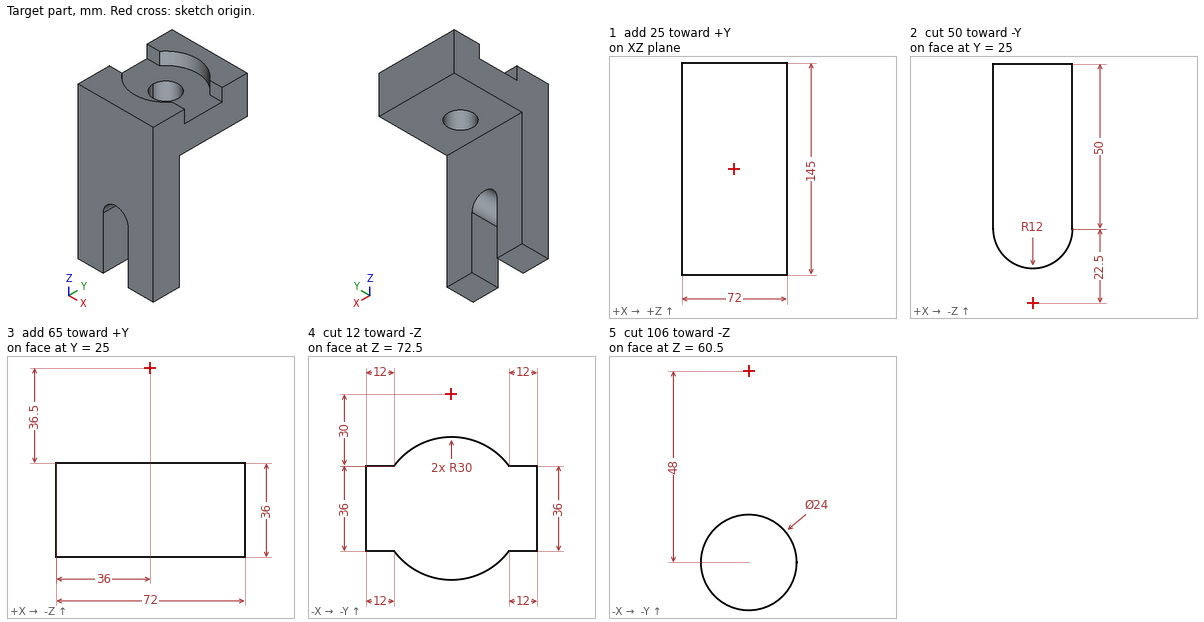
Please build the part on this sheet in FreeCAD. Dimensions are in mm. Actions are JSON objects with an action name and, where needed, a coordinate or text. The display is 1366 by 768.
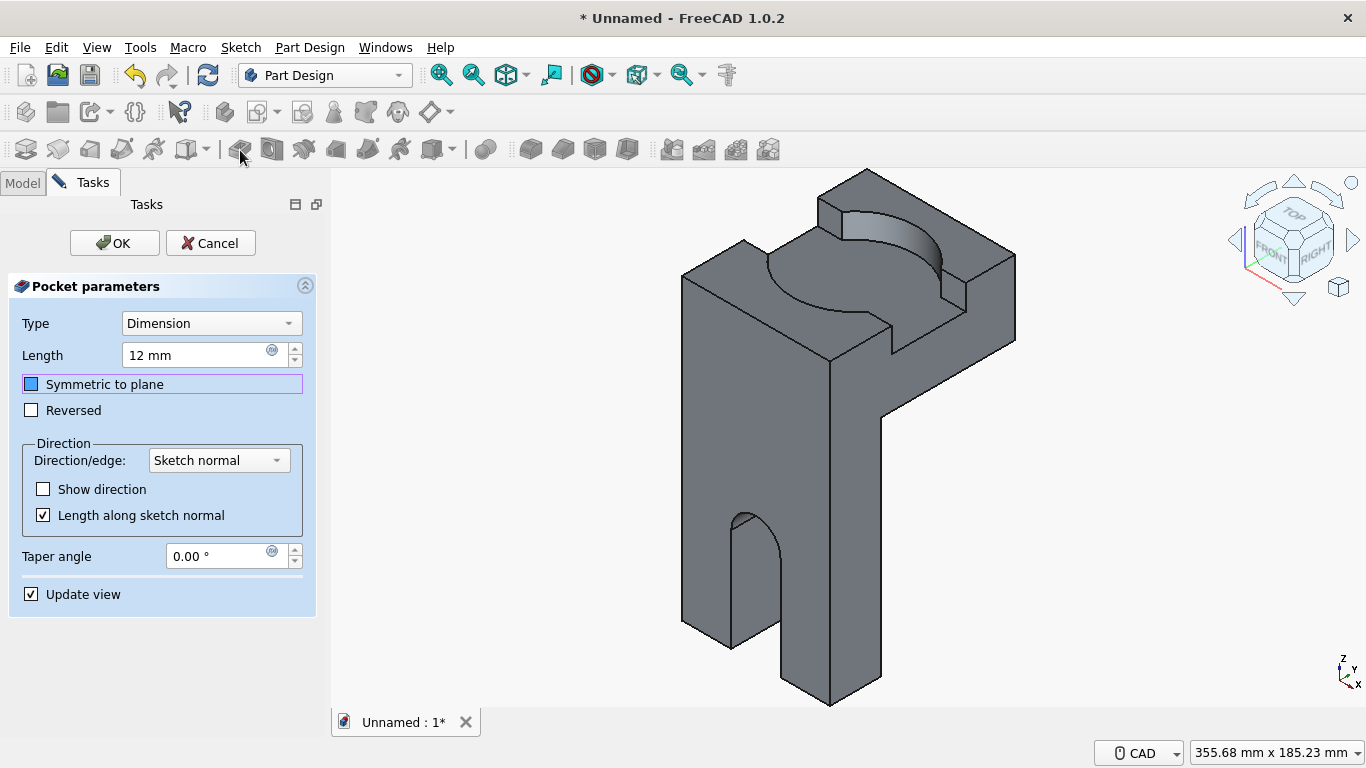
{"action": "left_click", "coordinate": [115, 243]}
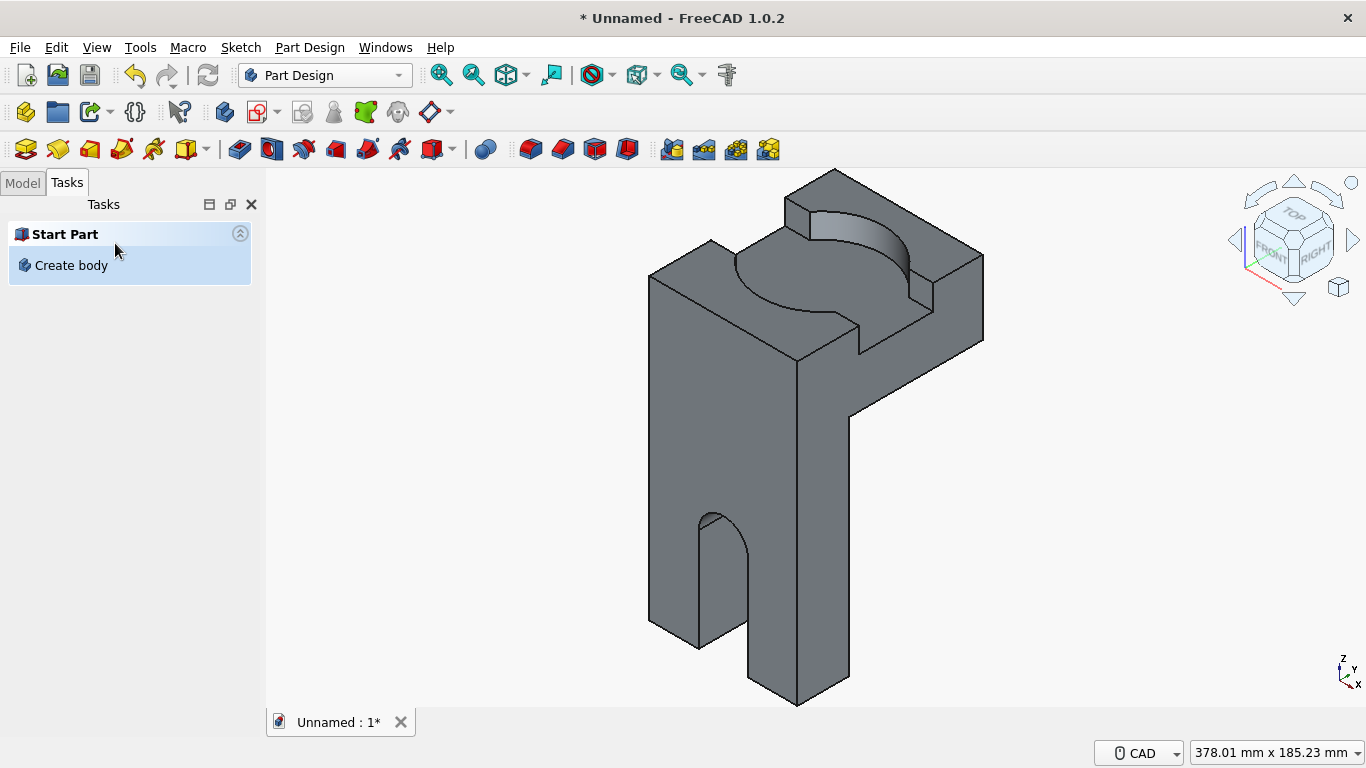
{"action": "left_click", "coordinate": [822, 289]}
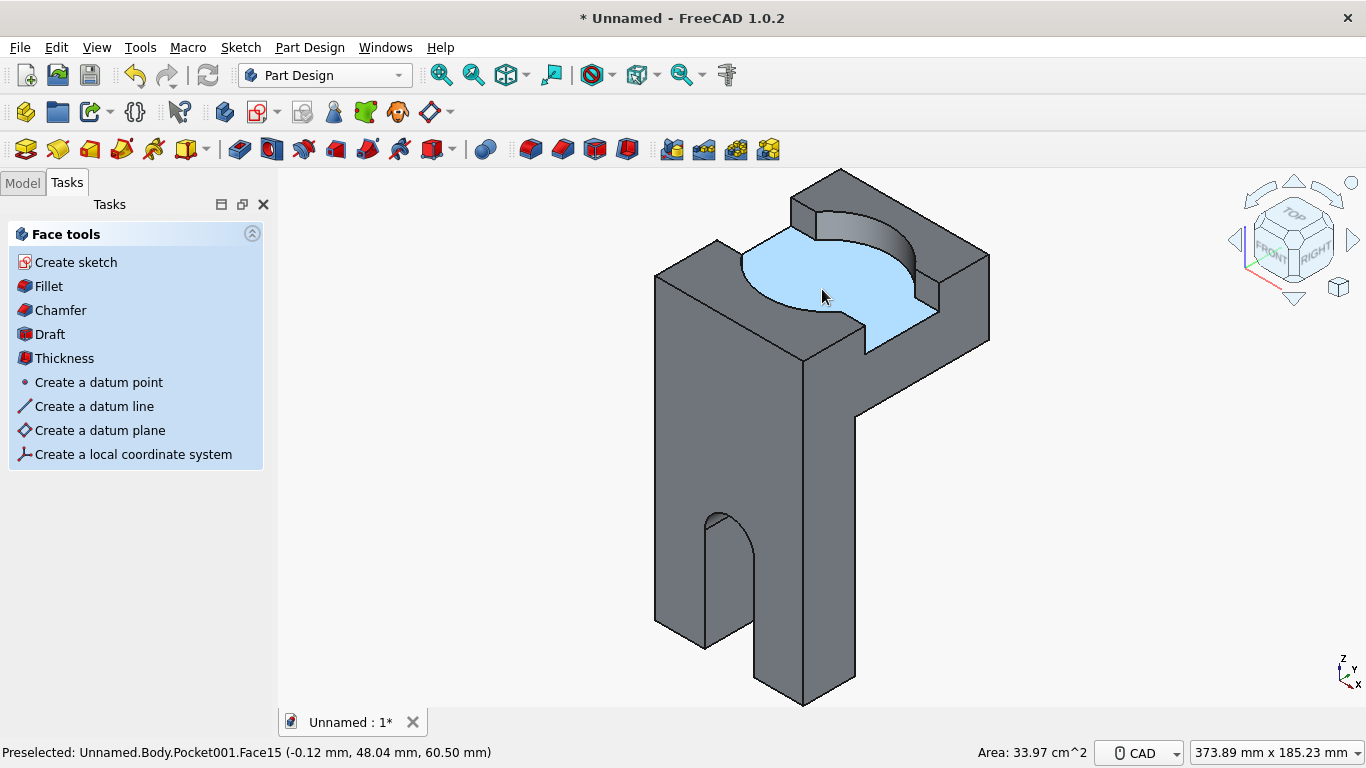
{"action": "left_click", "coordinate": [258, 112]}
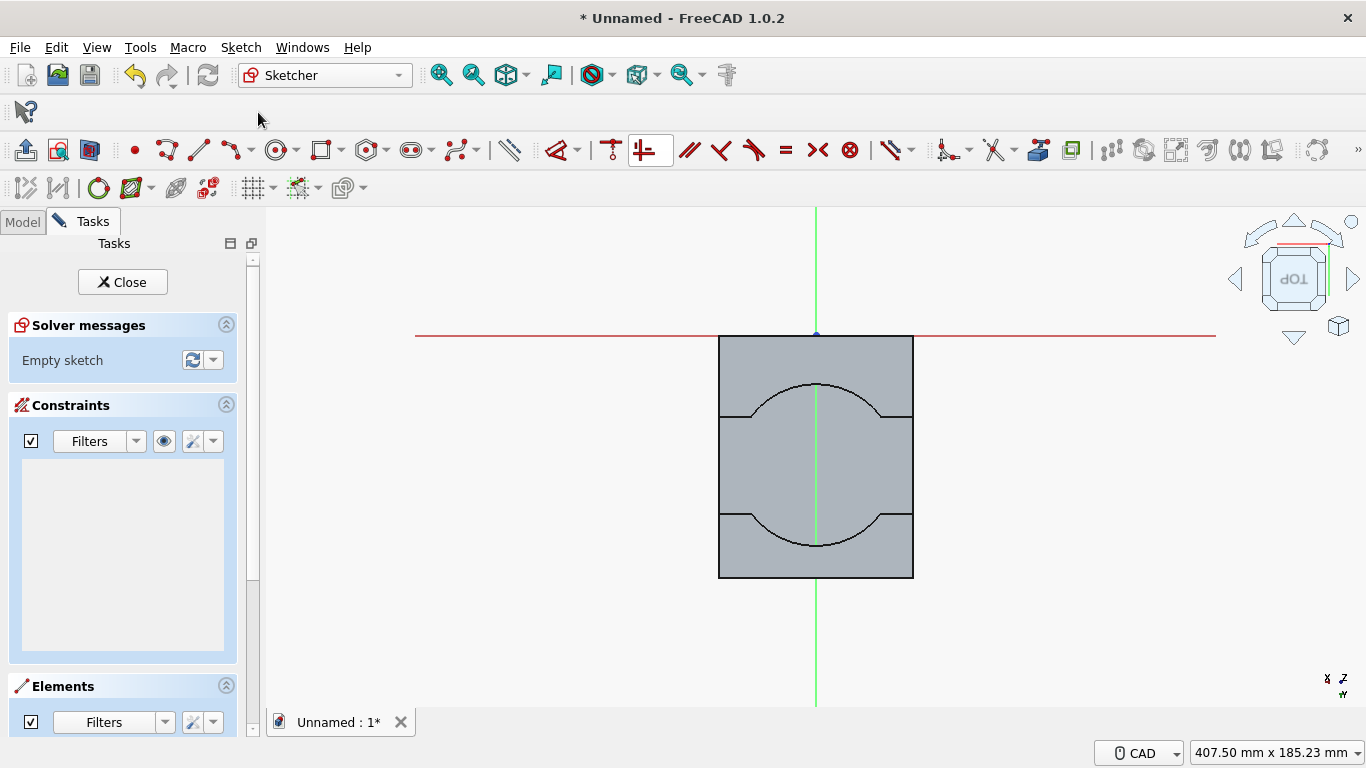
{"action": "scroll", "coordinate": [833, 467], "scroll_direction": "up", "scroll_amount": 8}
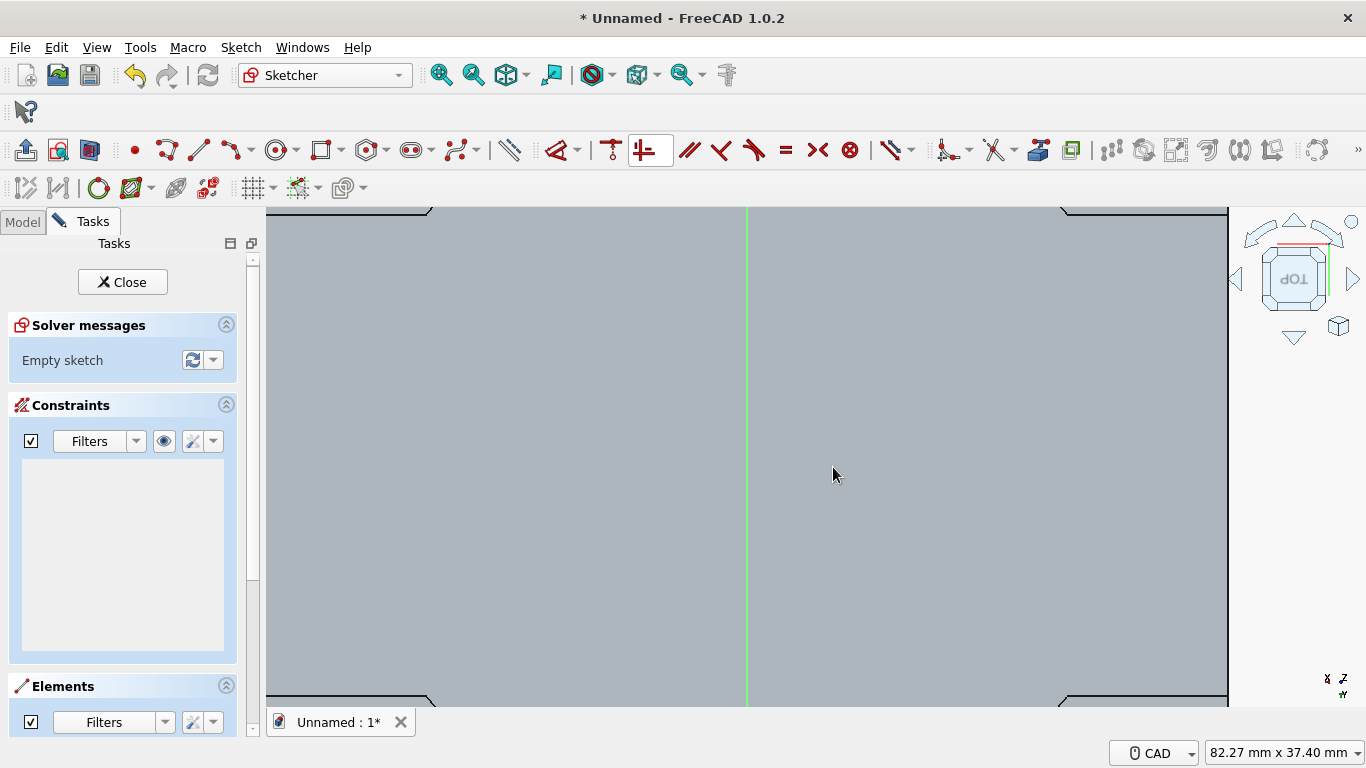
{"action": "left_click", "coordinate": [276, 150]}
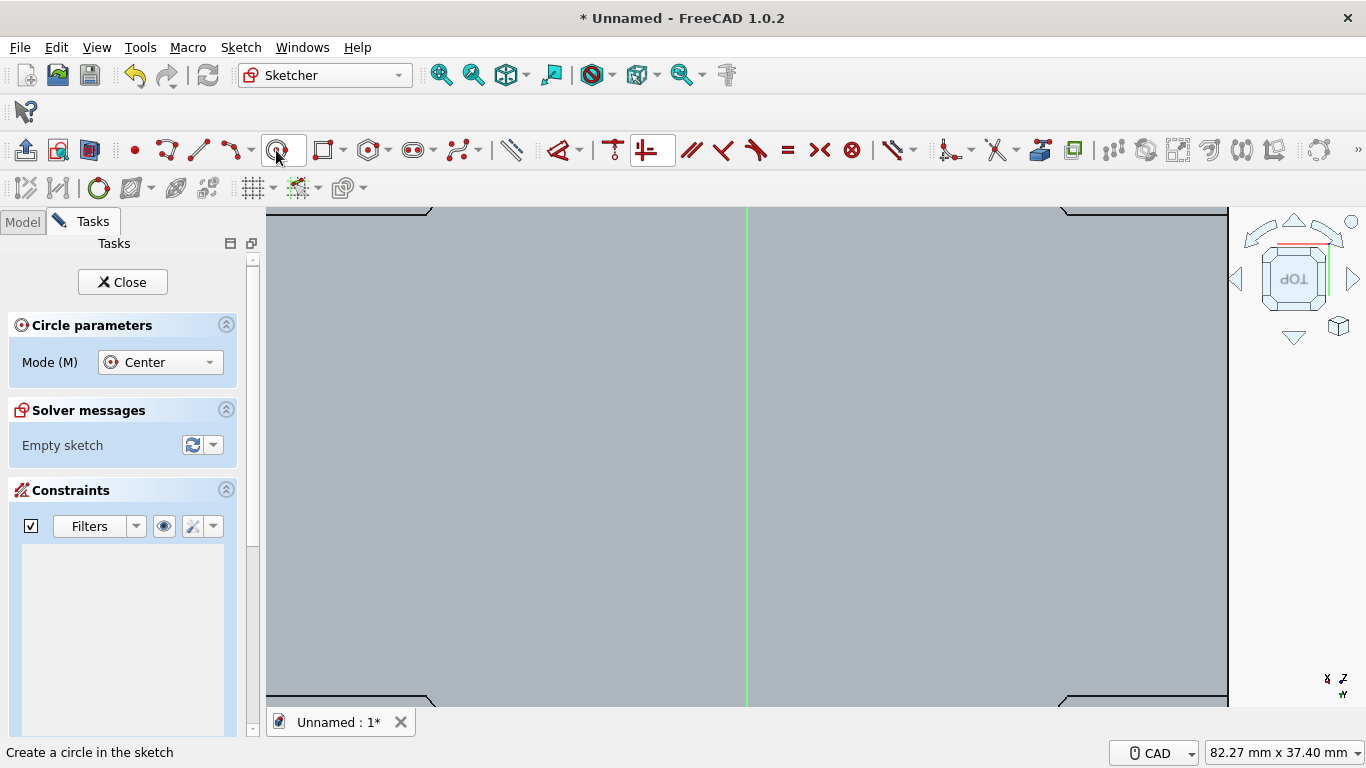
{"action": "left_click", "coordinate": [747, 456]}
{"action": "mouse_move", "coordinate": [860, 342]}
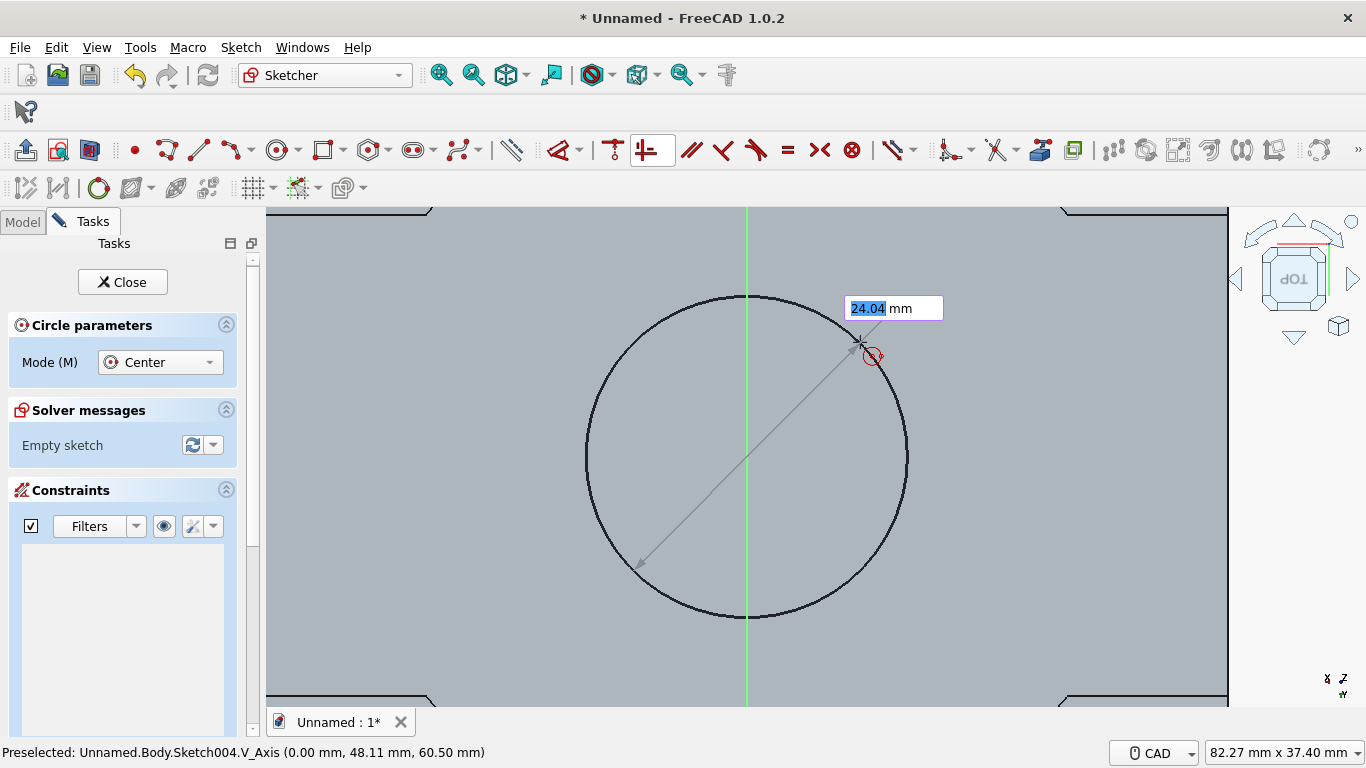
{"action": "type", "text": "24"}
{"action": "key", "text": "Return"}
{"action": "key", "text": "Escape"}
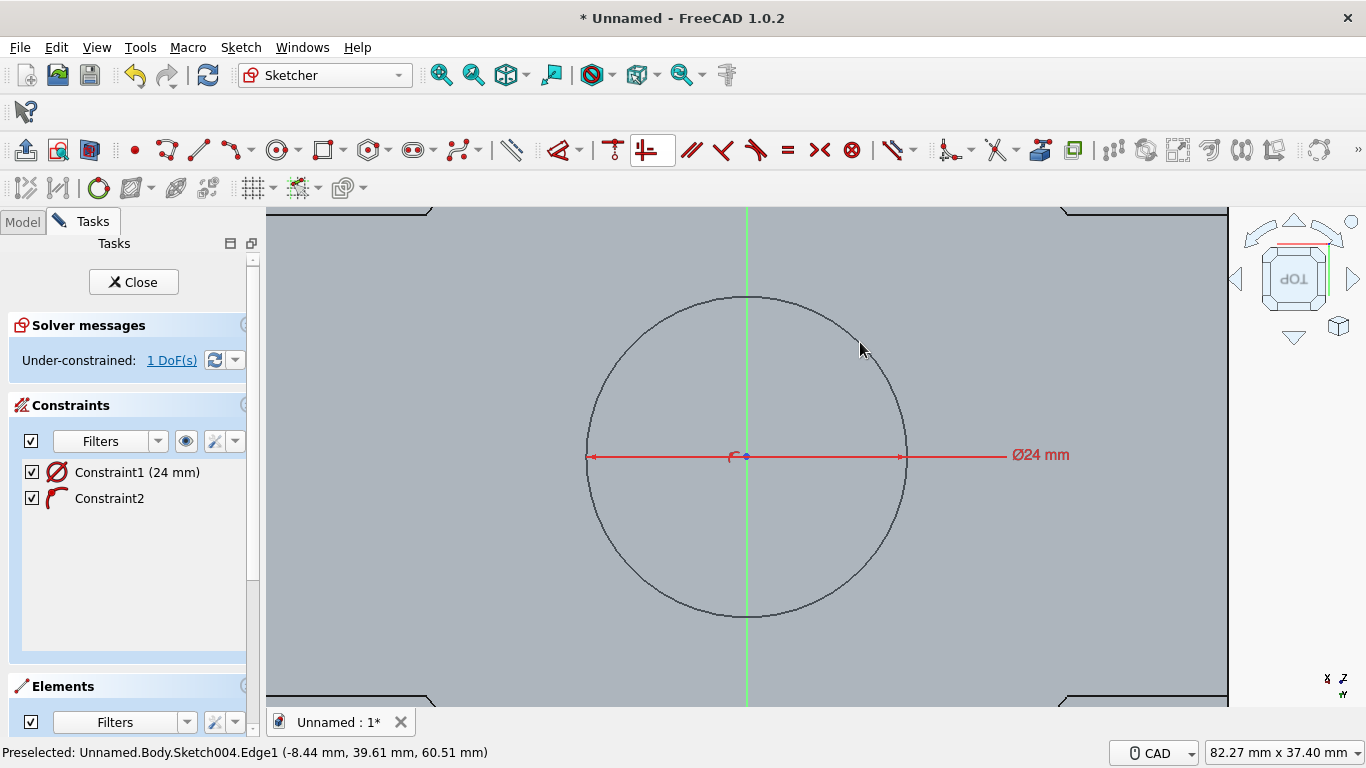
{"action": "left_click", "coordinate": [558, 150]}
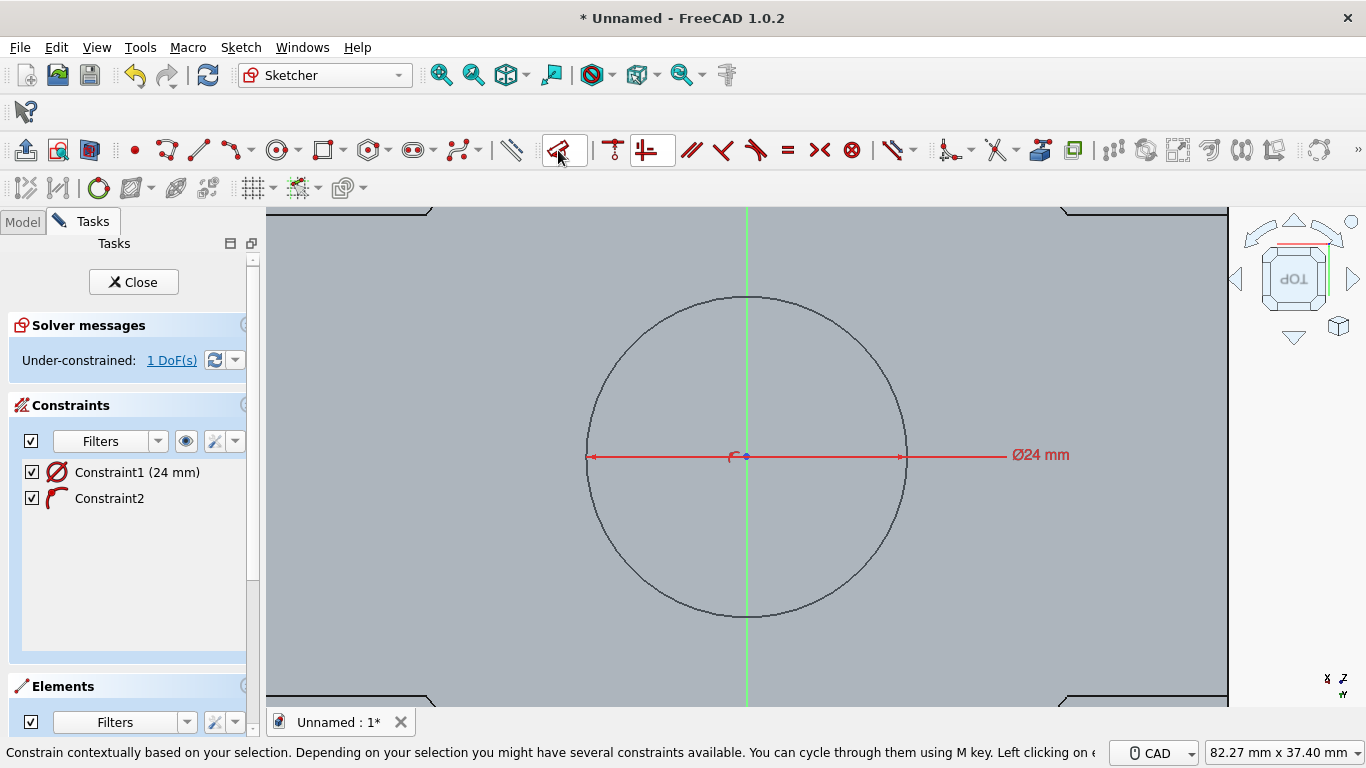
{"action": "left_click", "coordinate": [747, 457]}
{"action": "left_click", "coordinate": [781, 346]}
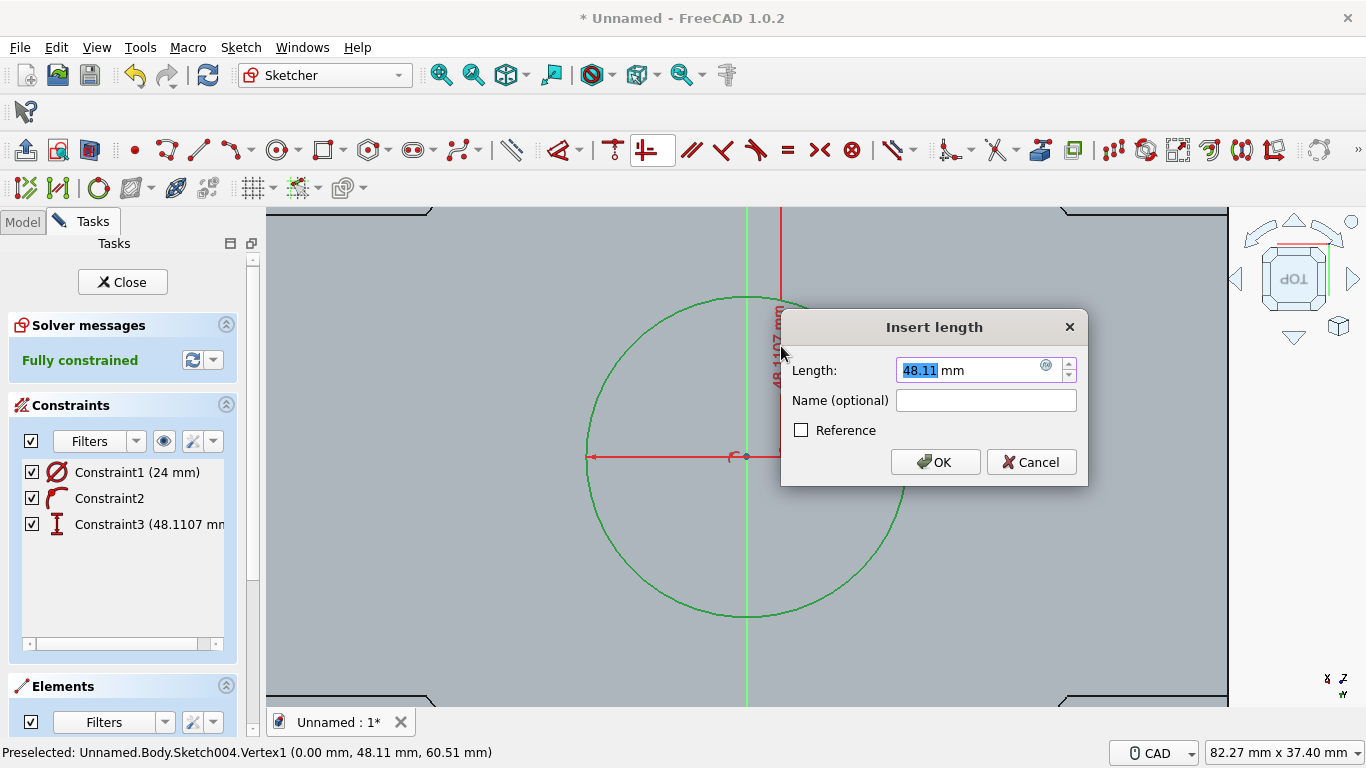
{"action": "type", "text": "48"}
{"action": "key", "text": "Return"}
{"action": "key", "text": "Escape"}